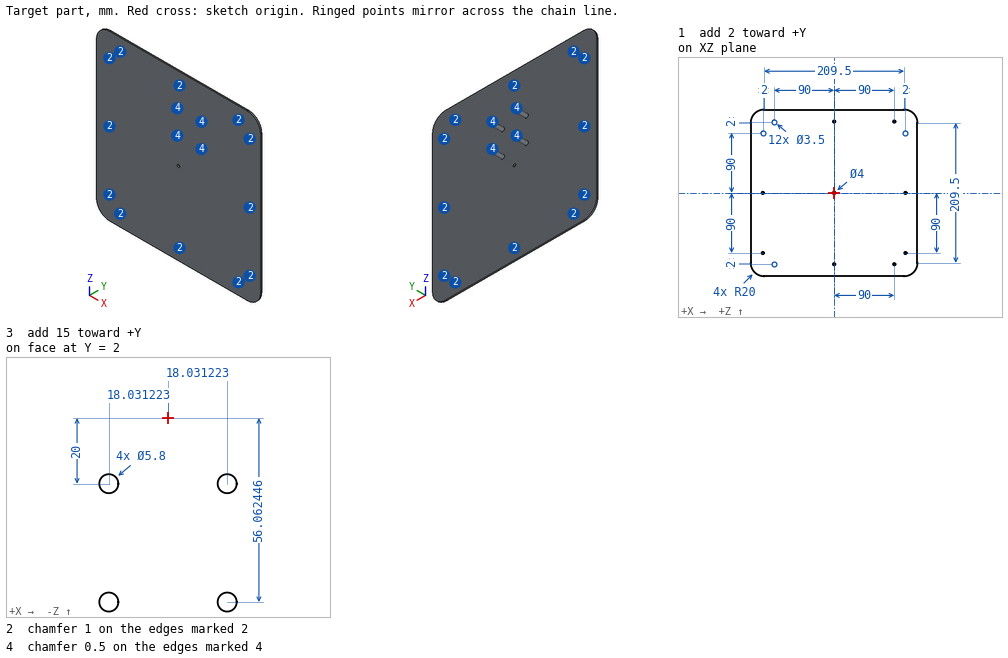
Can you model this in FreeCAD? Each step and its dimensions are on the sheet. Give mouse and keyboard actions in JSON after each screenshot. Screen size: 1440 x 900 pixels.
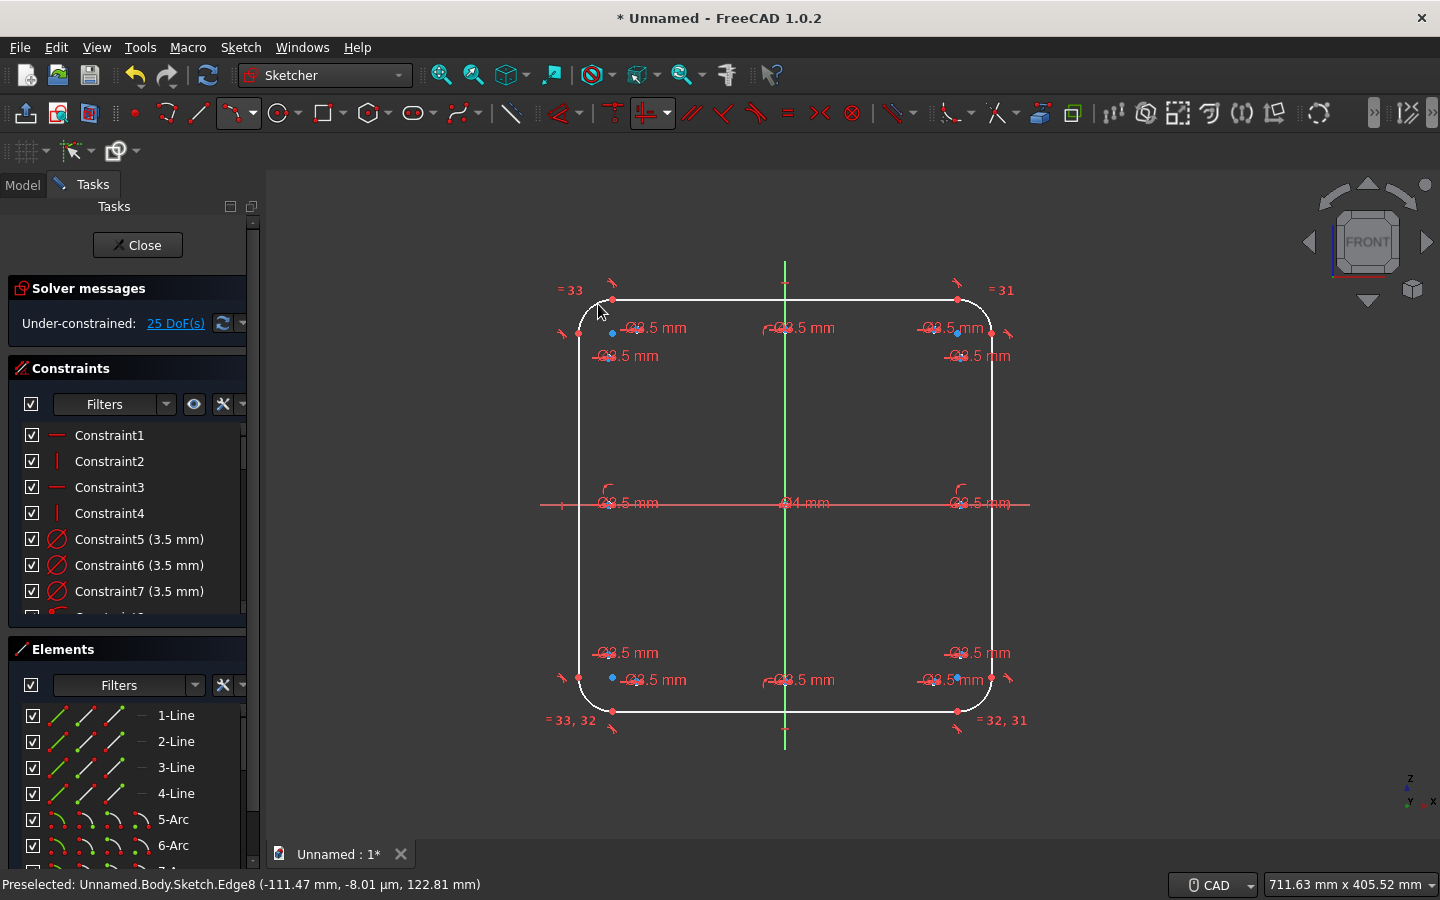
{"action": "left_click", "coordinate": [637, 330]}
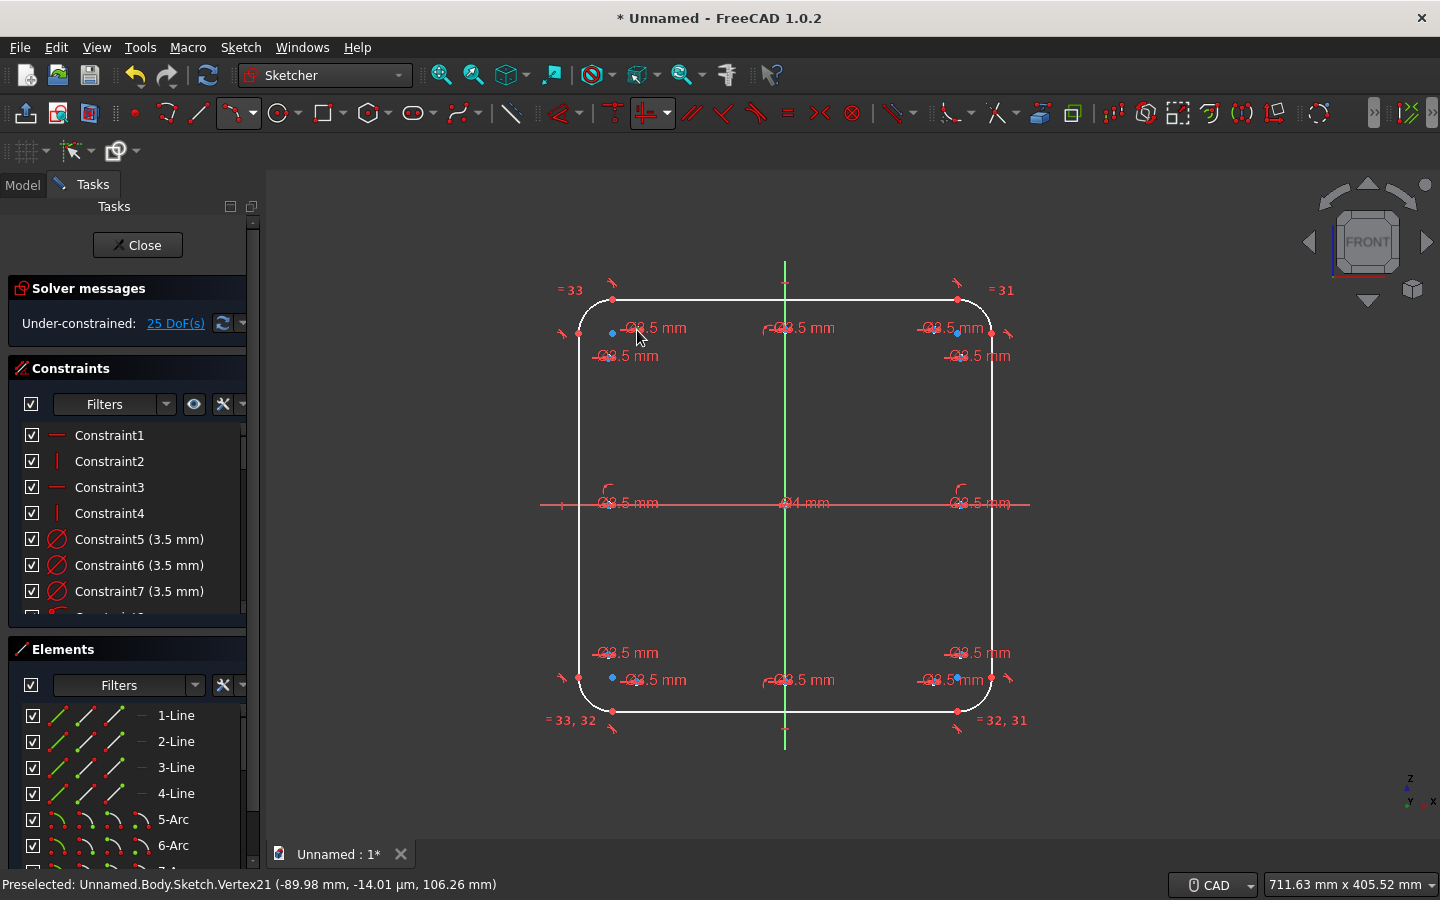
{"action": "left_click", "coordinate": [785, 330]}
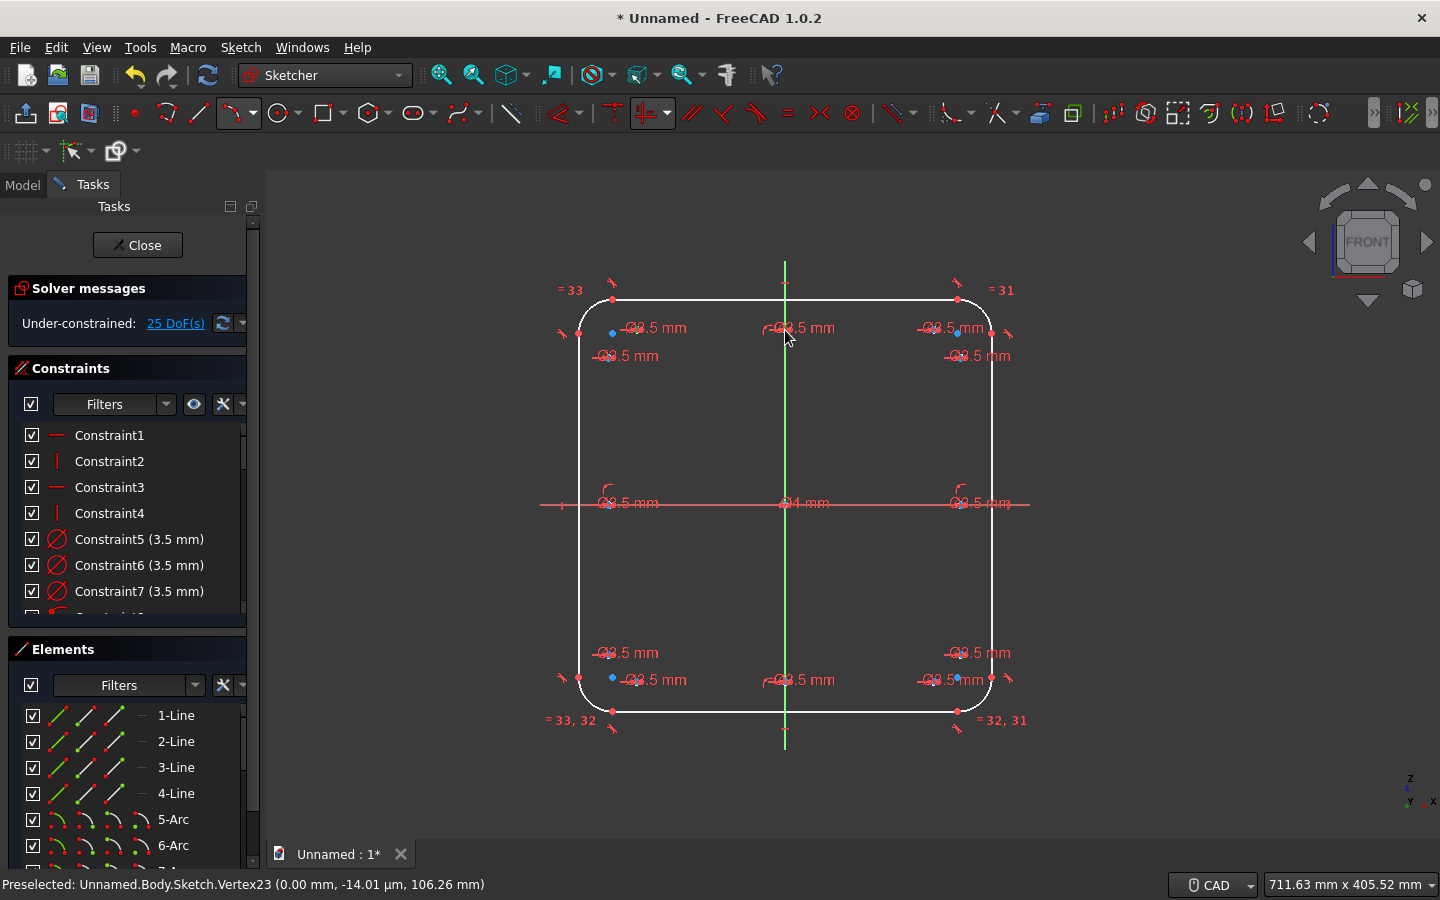
{"action": "key", "text": "h"}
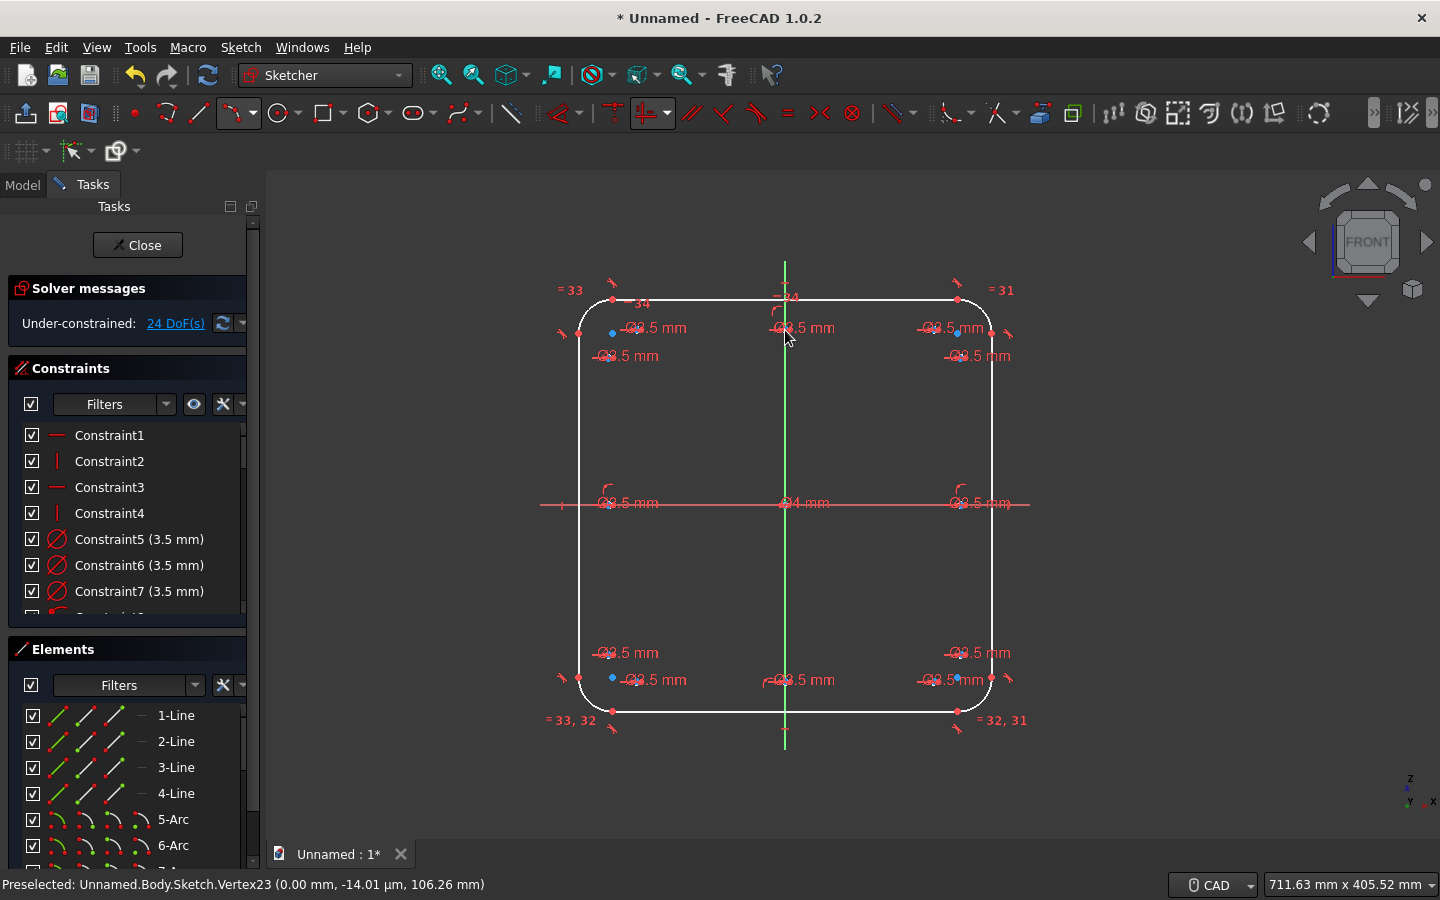
{"action": "left_click", "coordinate": [785, 330]}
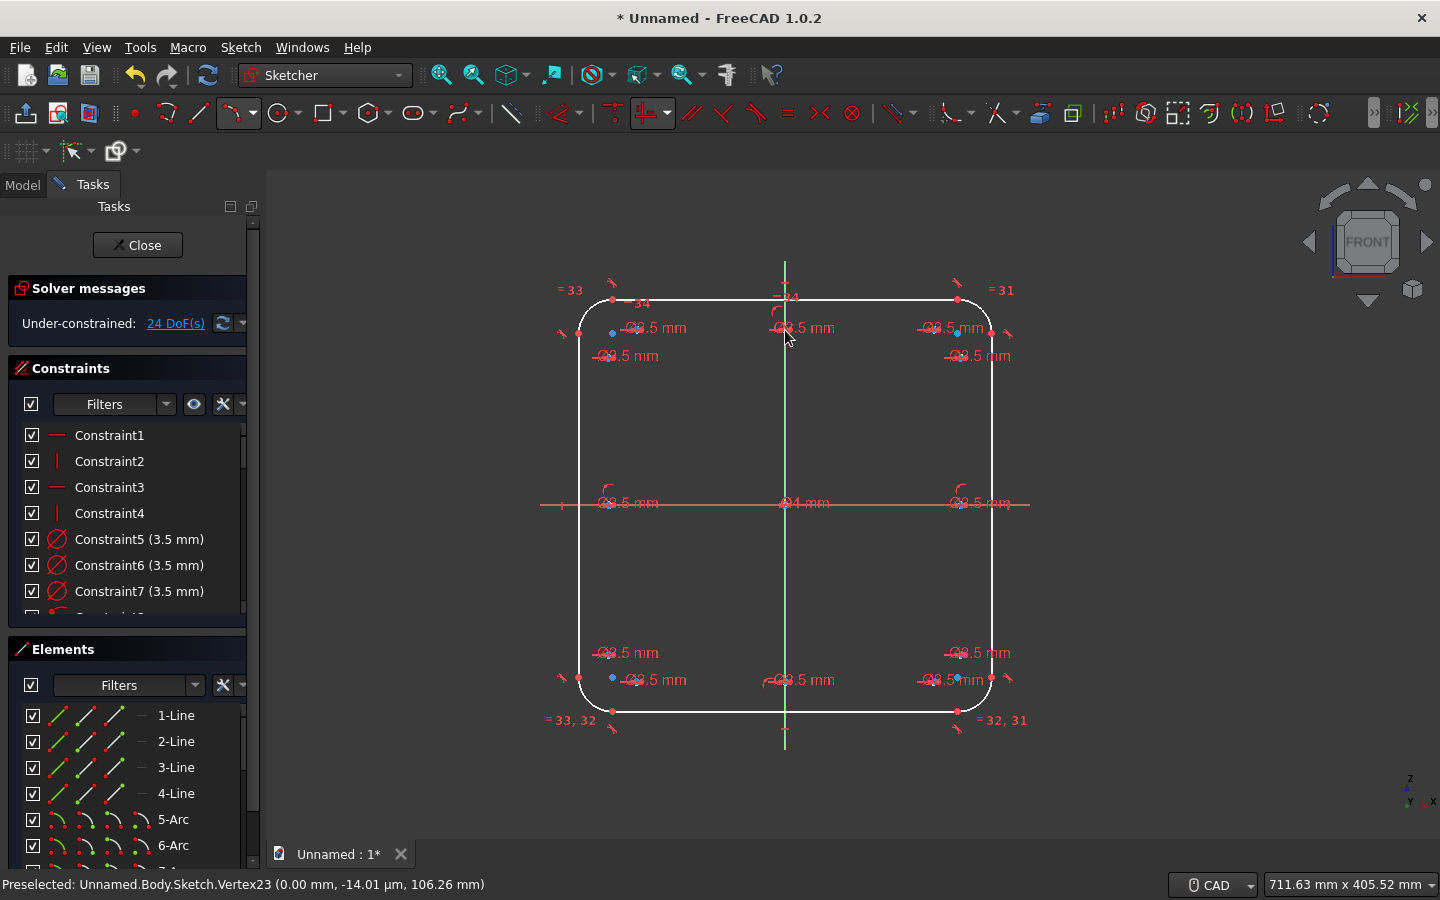
{"action": "left_click", "coordinate": [934, 330]}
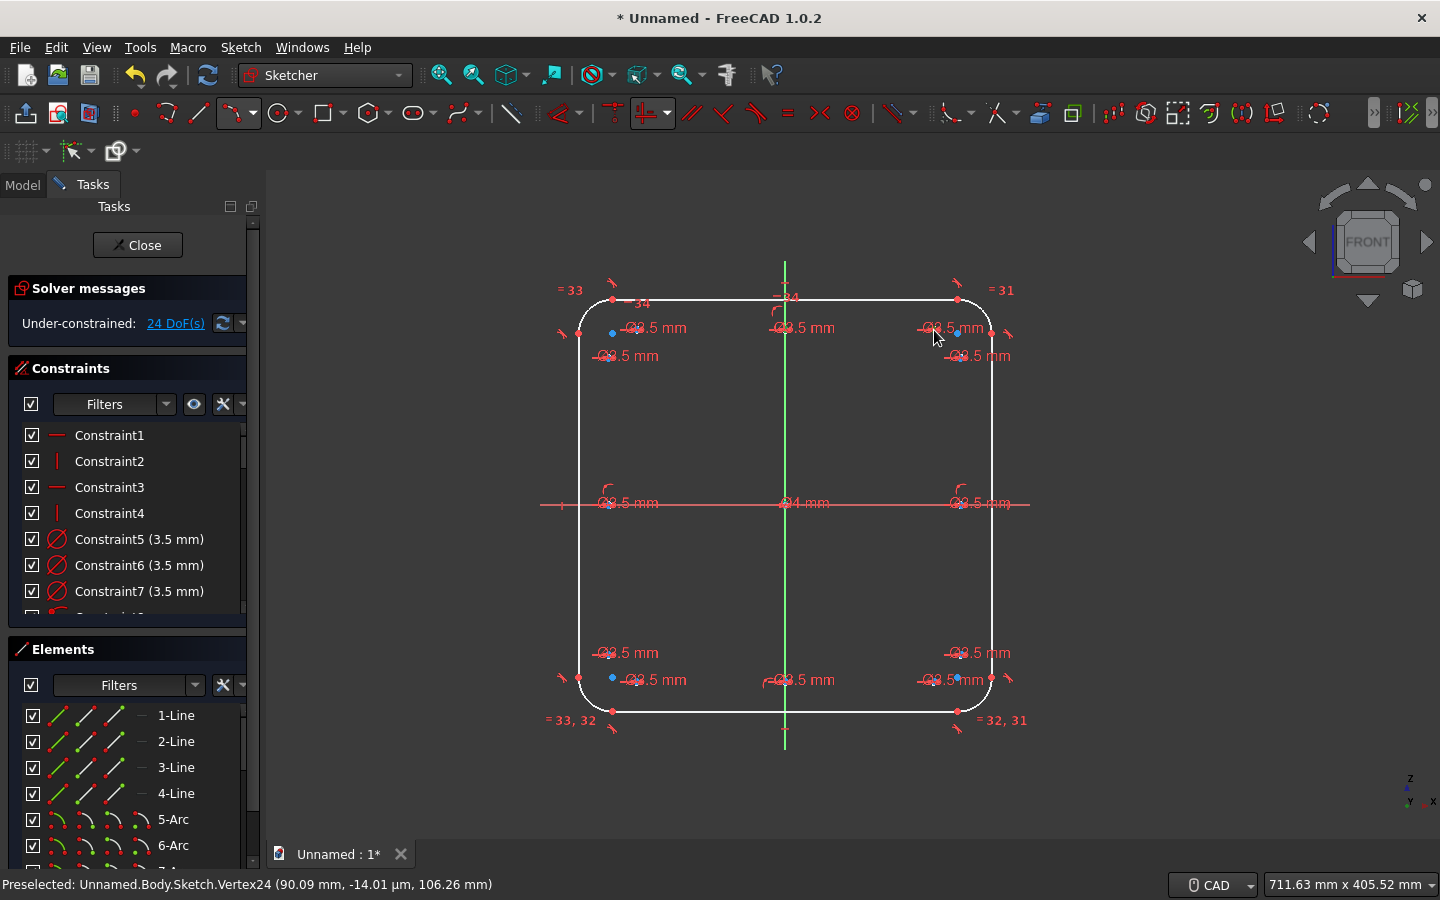
{"action": "left_click", "coordinate": [670, 114]}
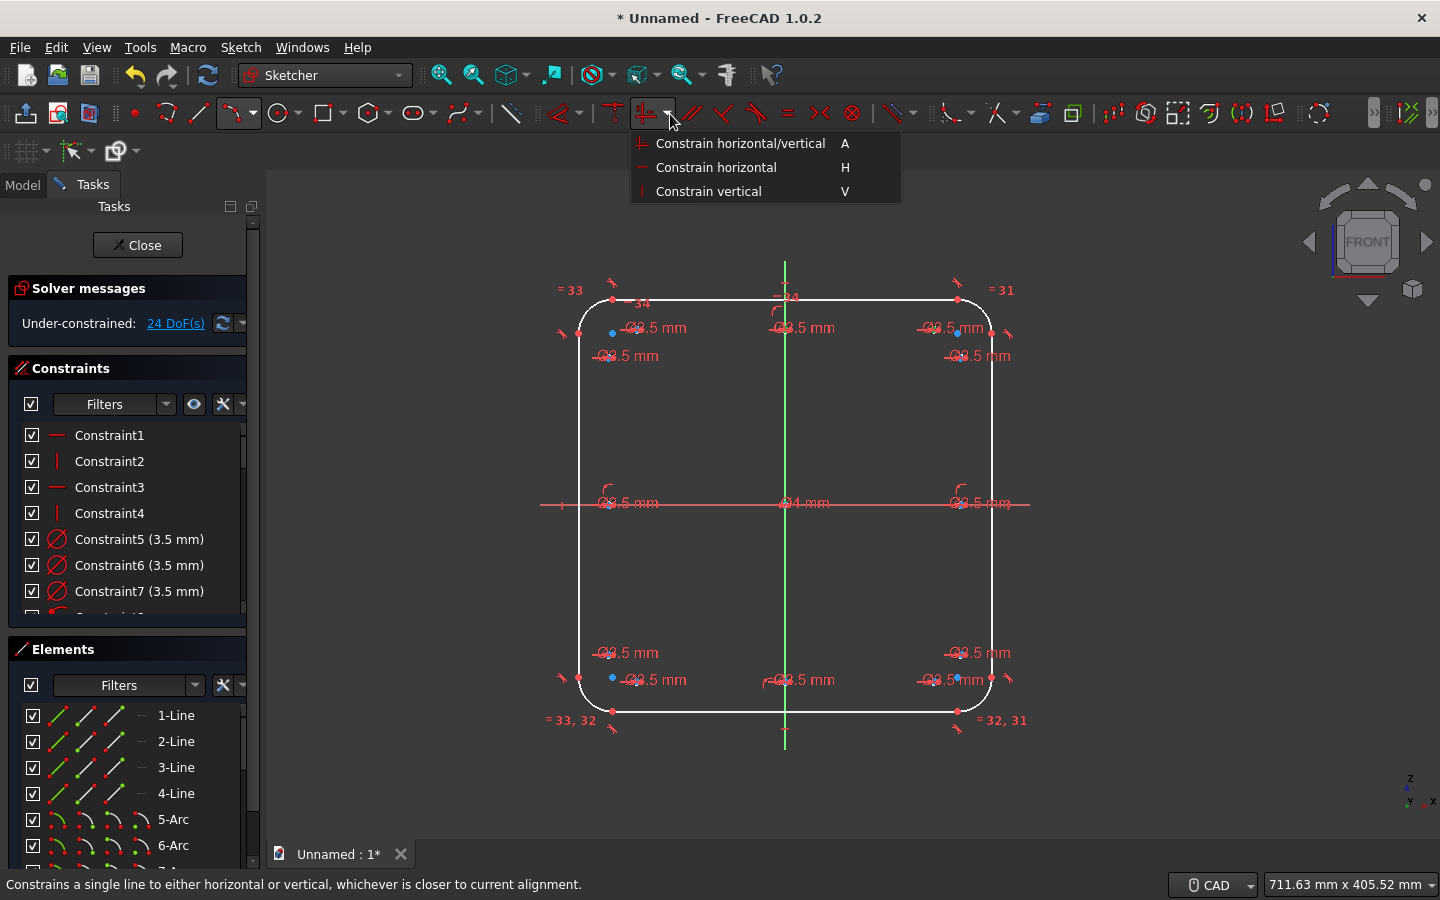
{"action": "left_click", "coordinate": [766, 167]}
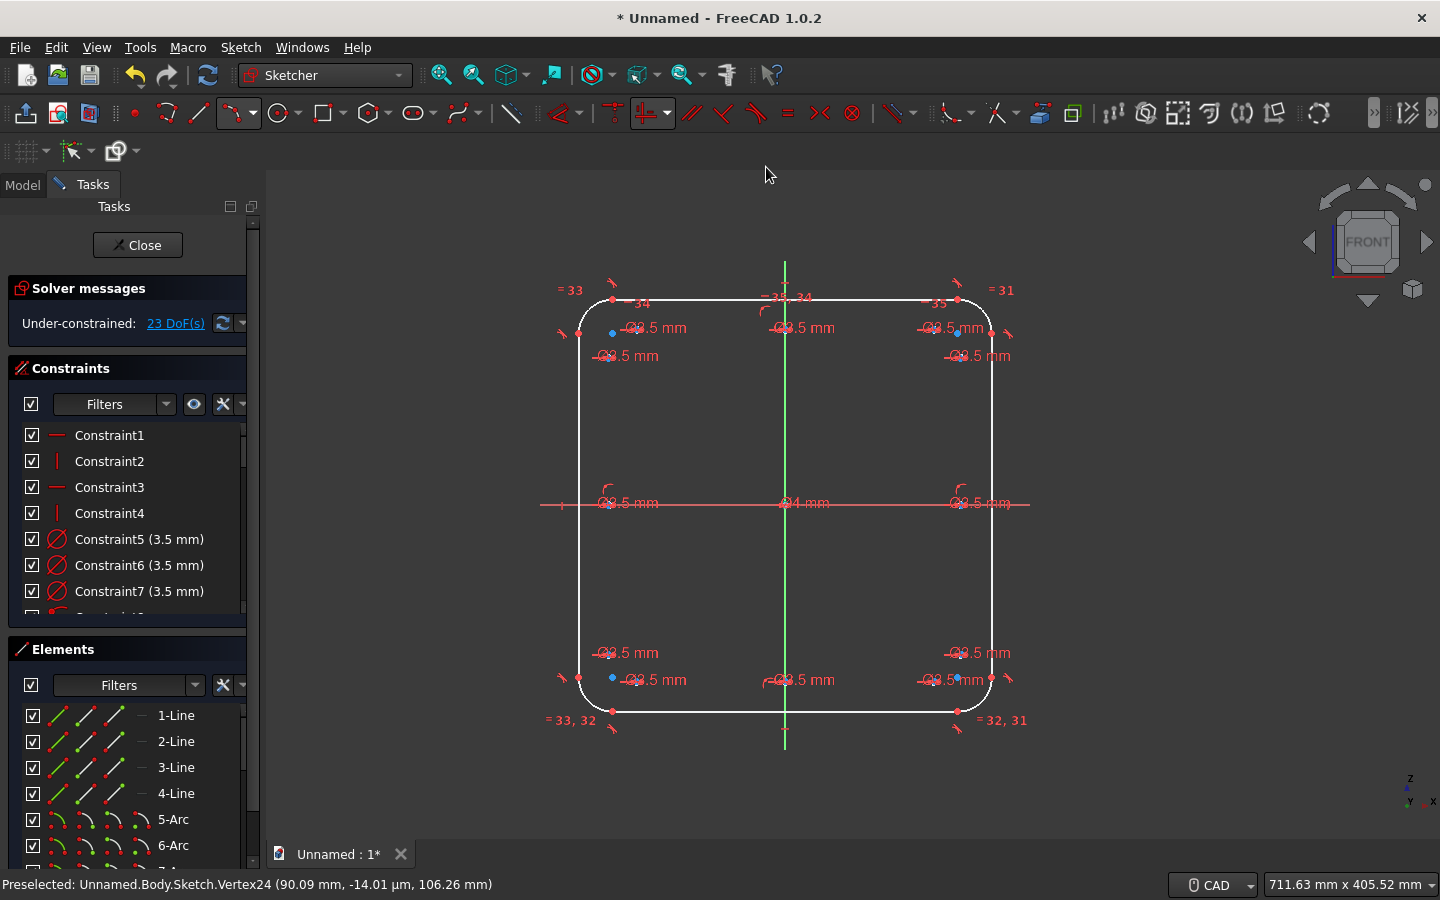
{"action": "left_click", "coordinate": [609, 358]}